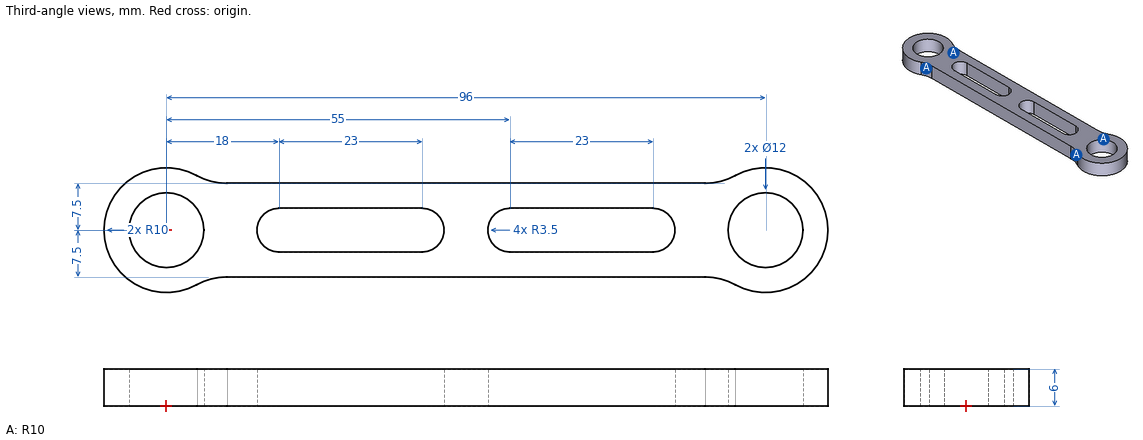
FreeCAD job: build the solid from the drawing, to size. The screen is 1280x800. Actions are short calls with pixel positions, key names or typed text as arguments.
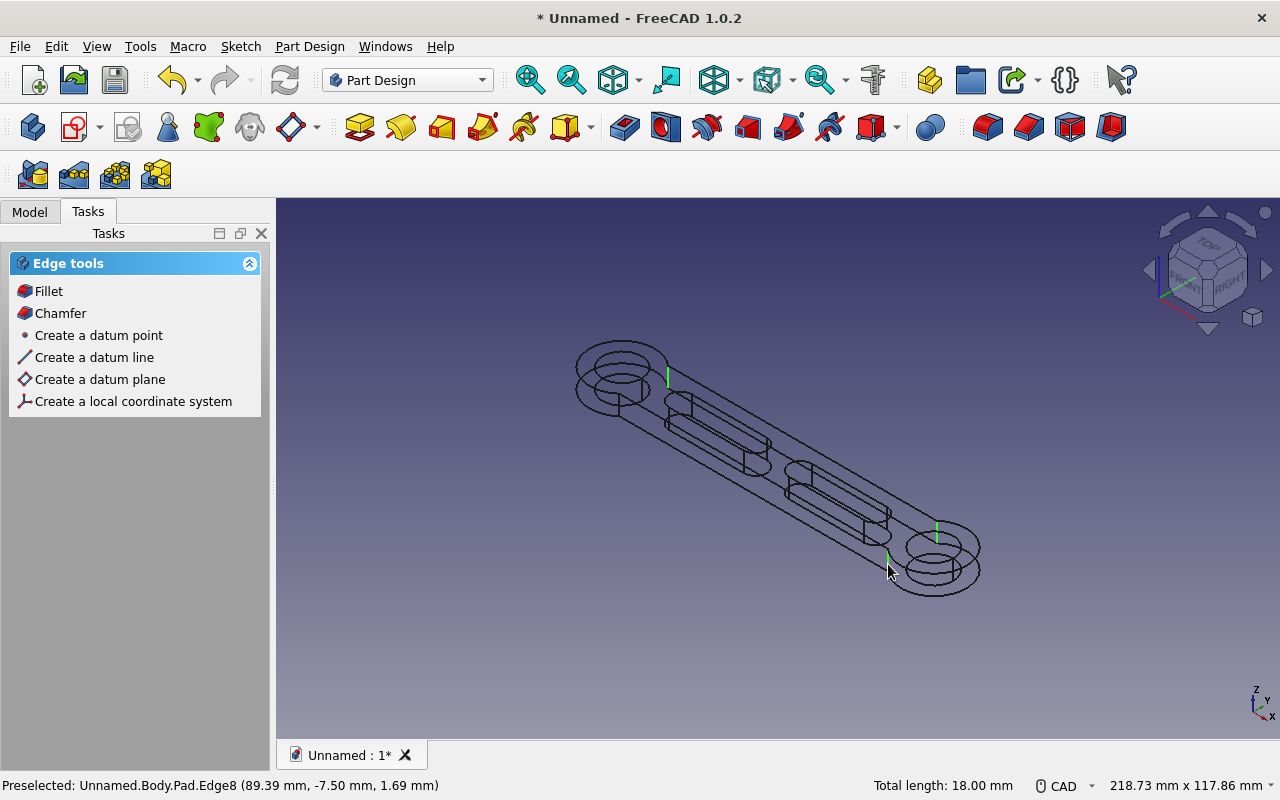
click(619, 404, ctrl)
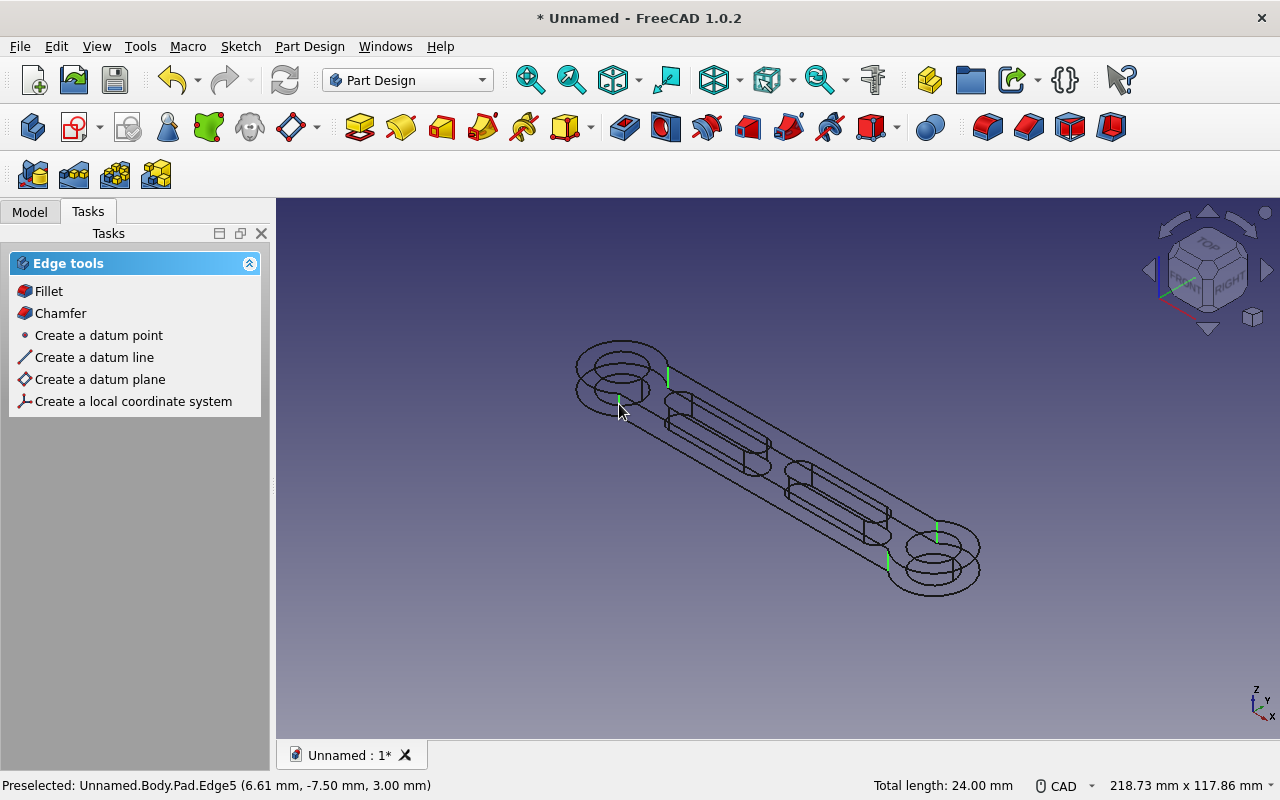
key(v)
key(1)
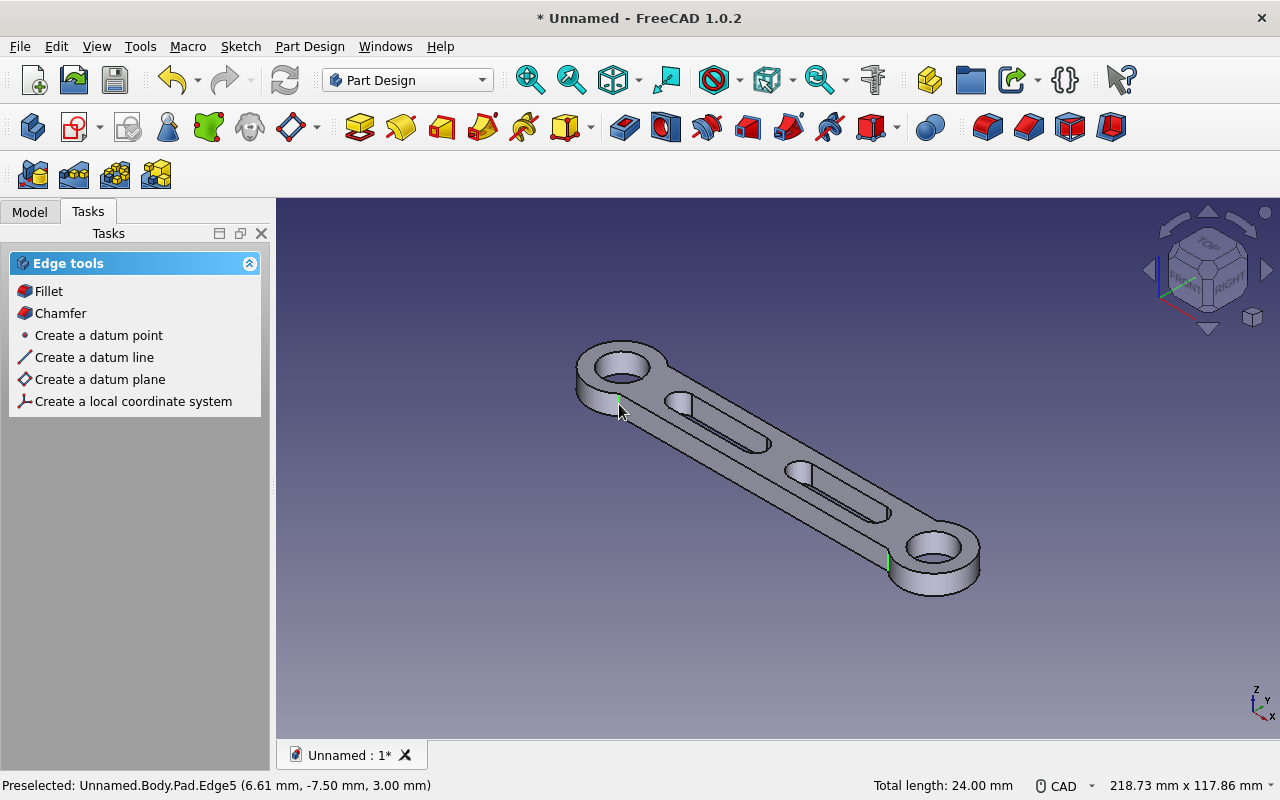
click(988, 128)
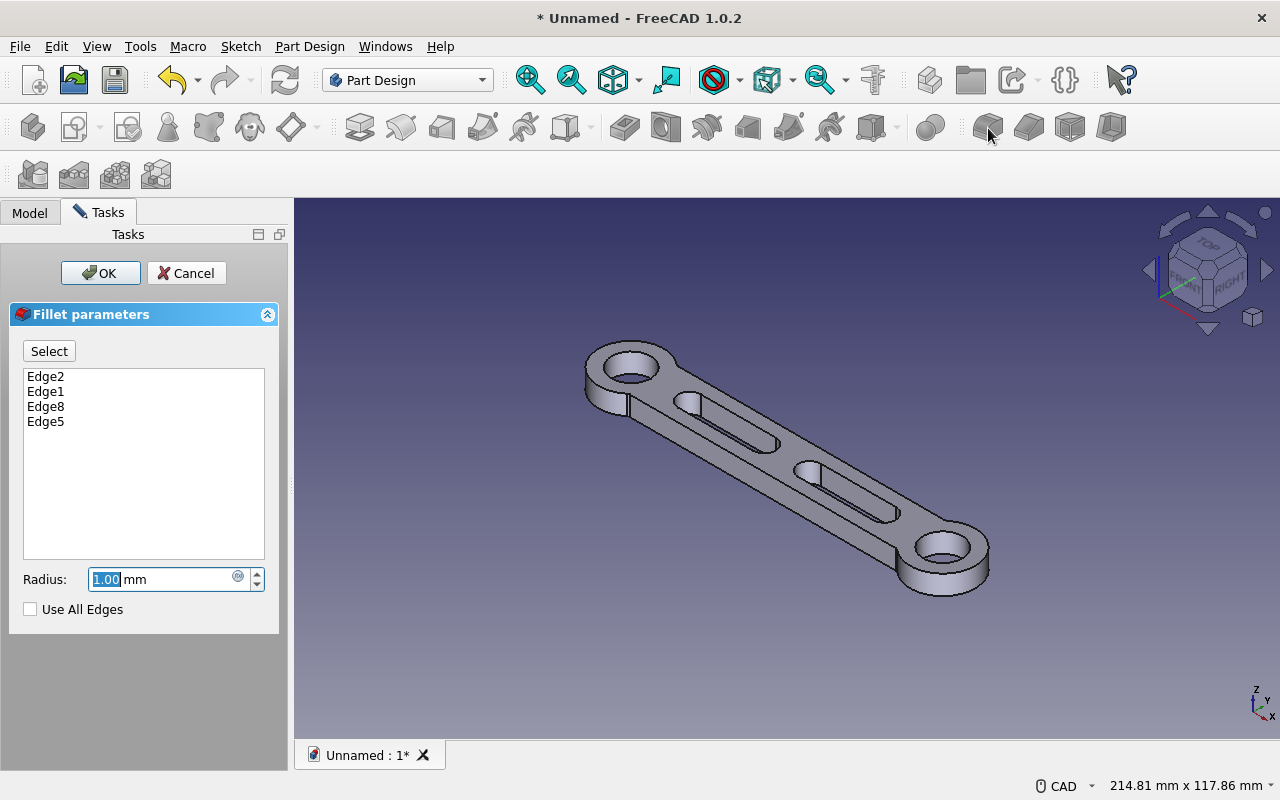
text(10)
key(Tab)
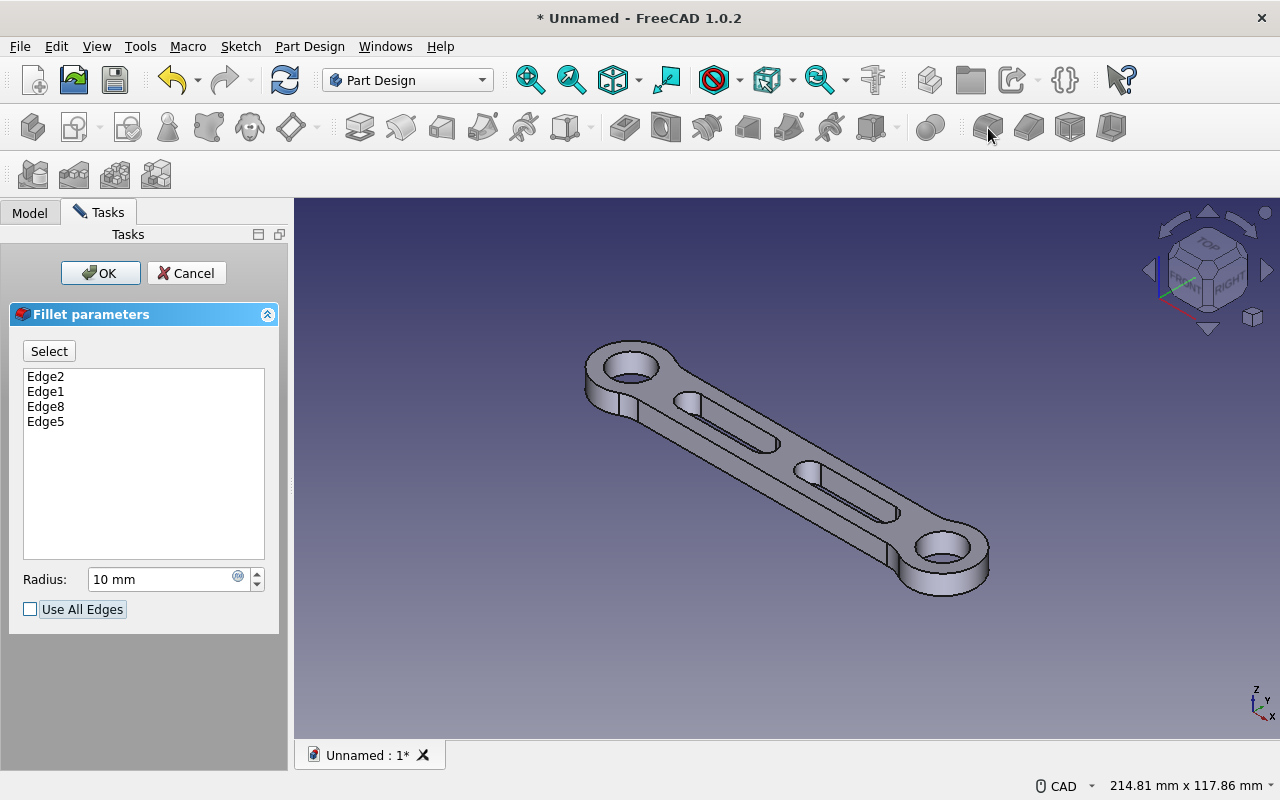
click(101, 273)